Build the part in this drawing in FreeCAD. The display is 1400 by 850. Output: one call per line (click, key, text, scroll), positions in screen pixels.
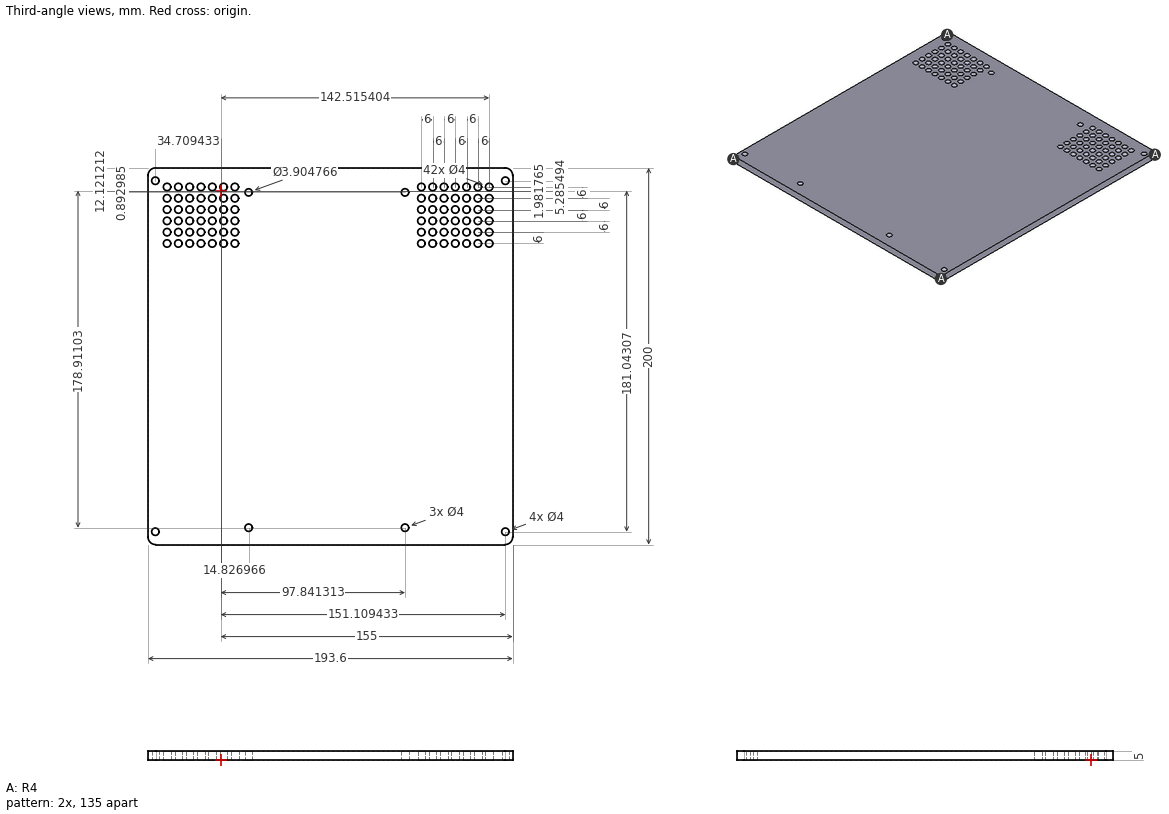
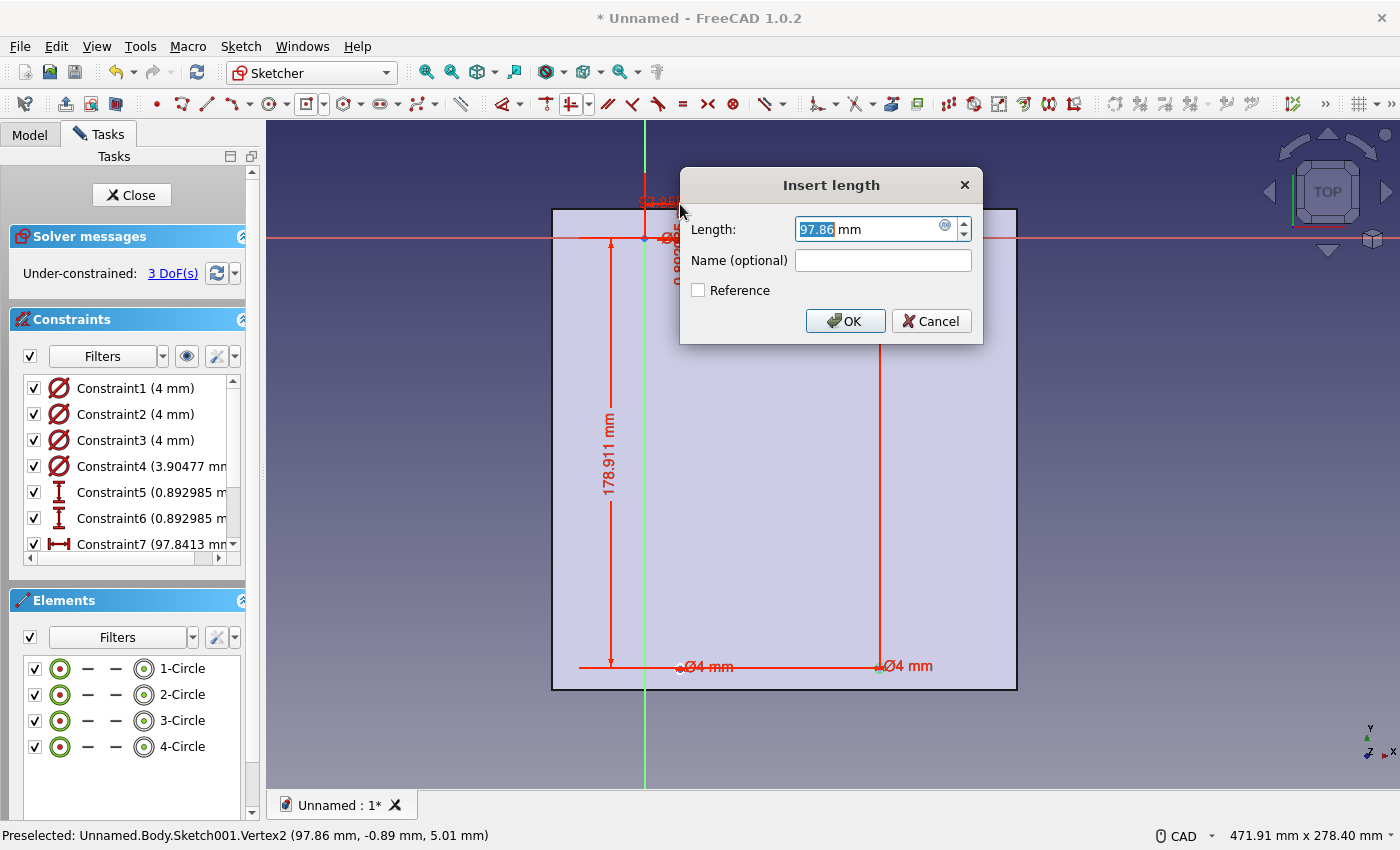
text(97.841313)
key(Return)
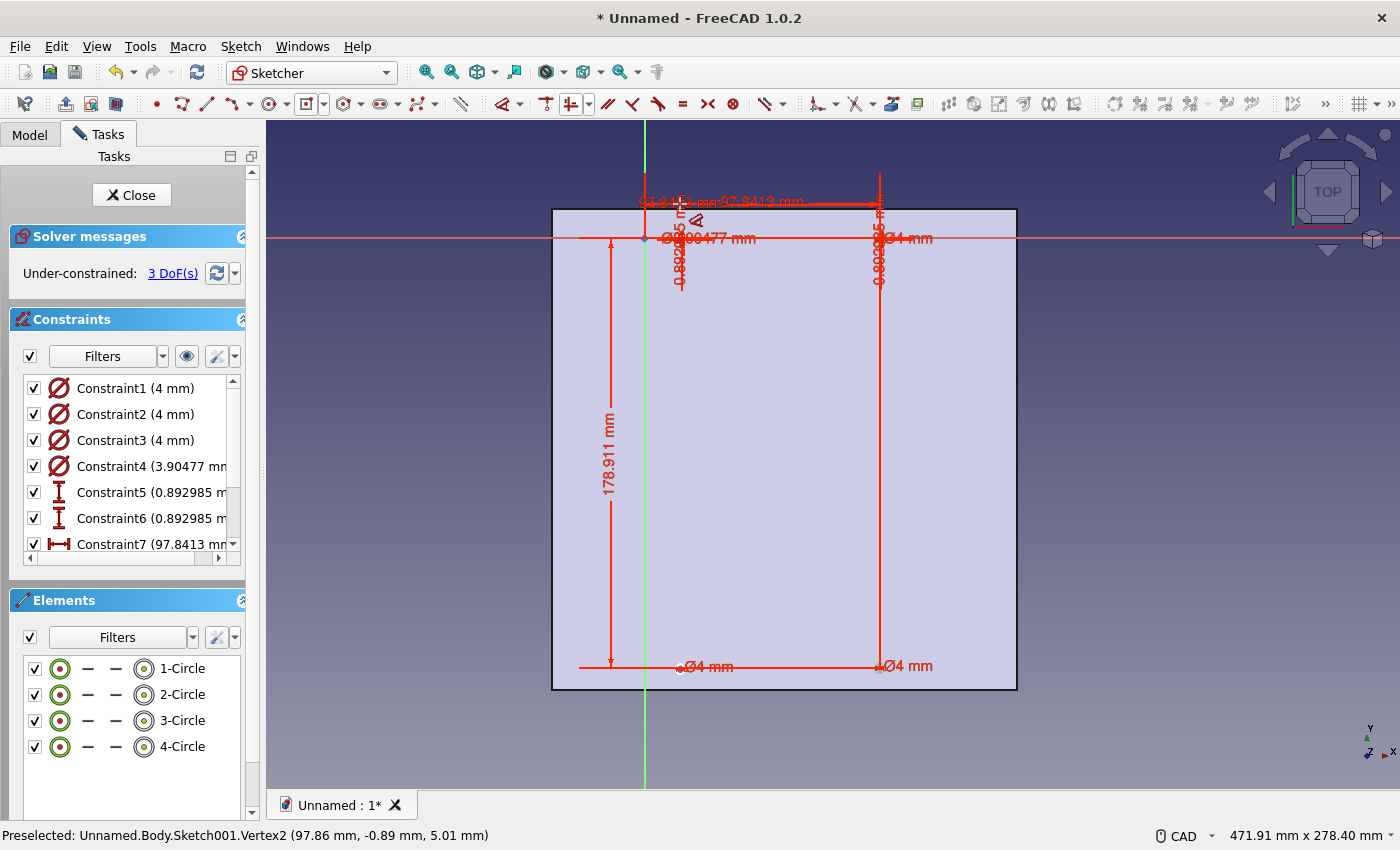
click(680, 669)
click(662, 703)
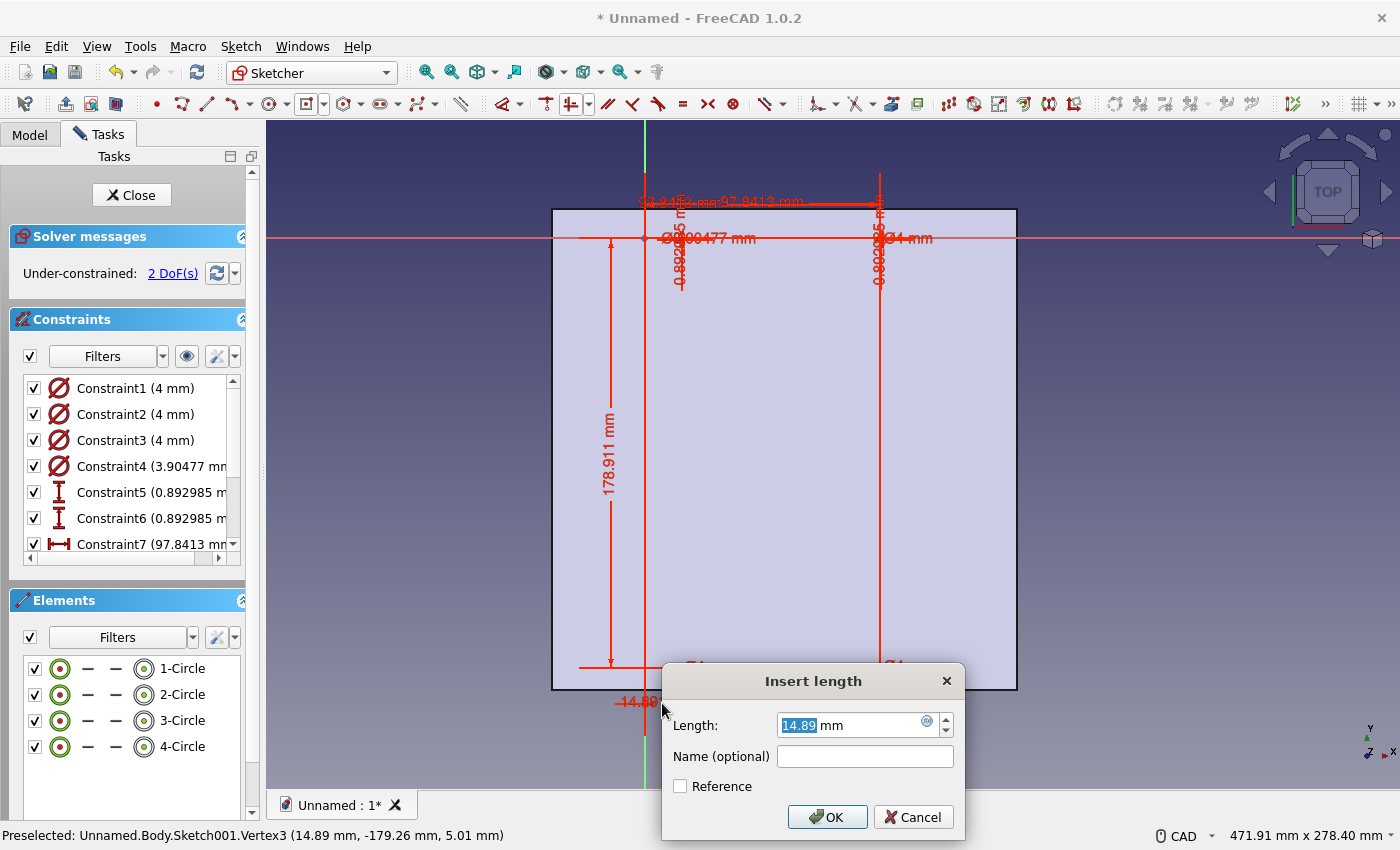
text(14.826966)
key(Return)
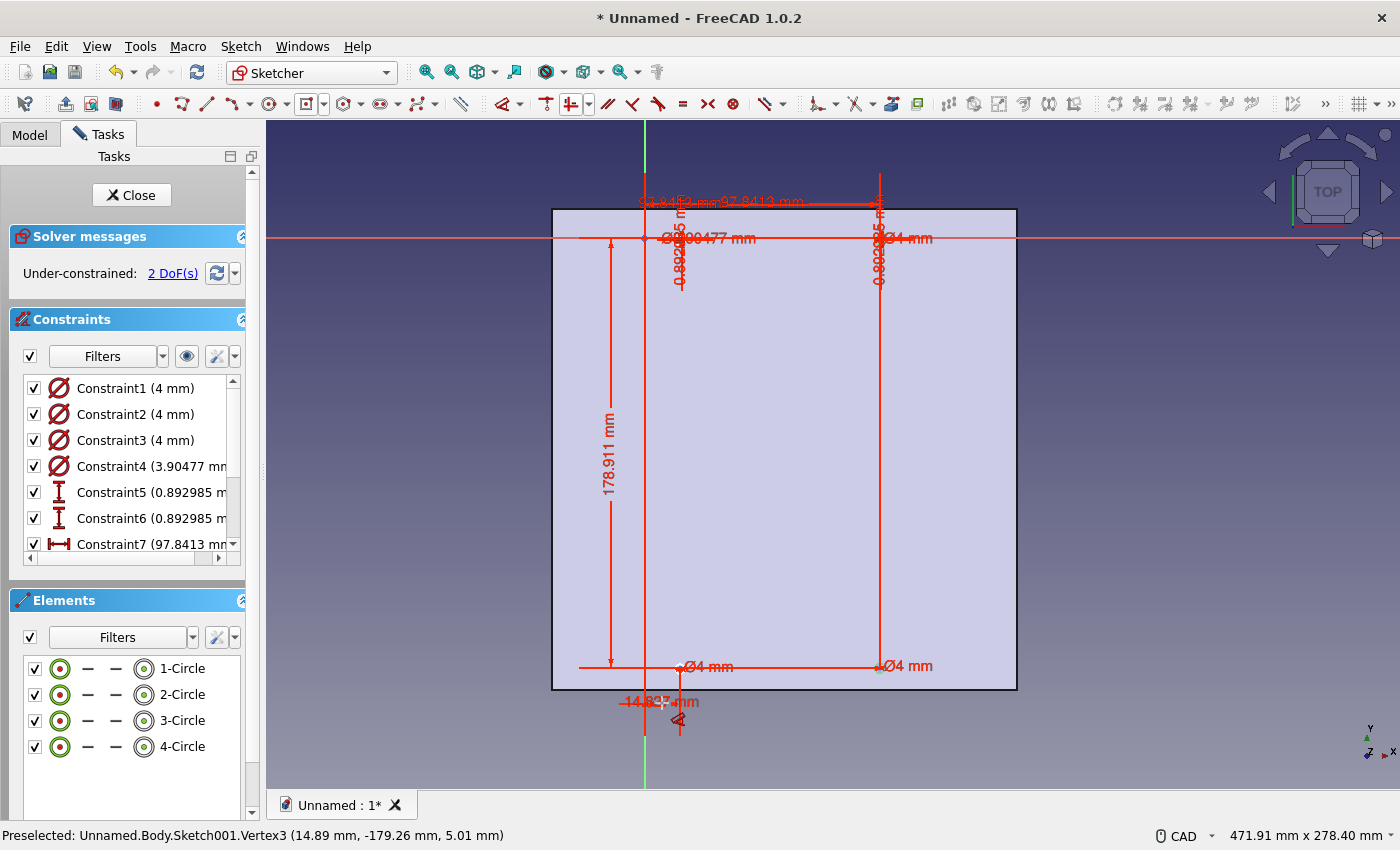
click(680, 669)
click(611, 355)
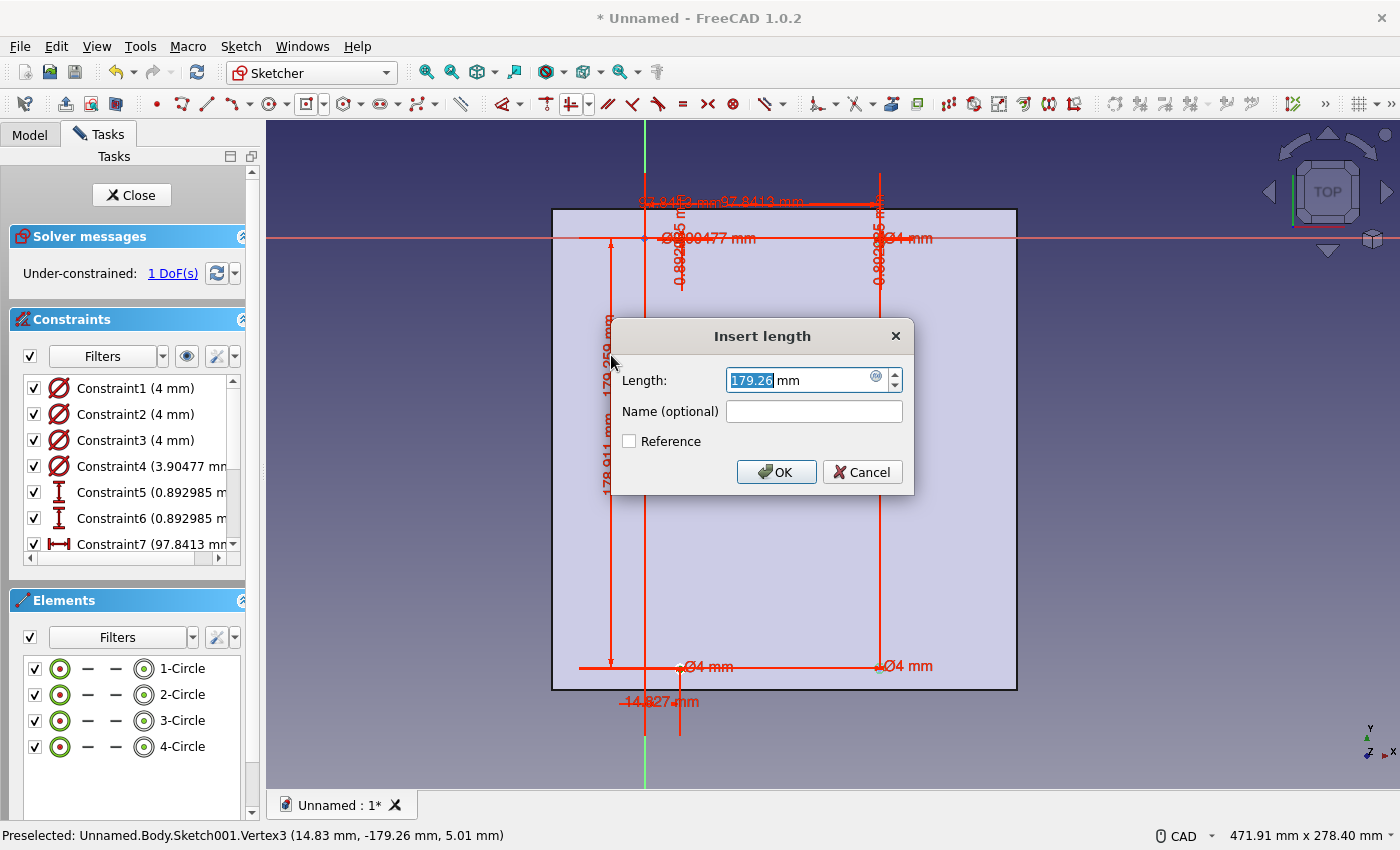
text(178.91103)
key(Return)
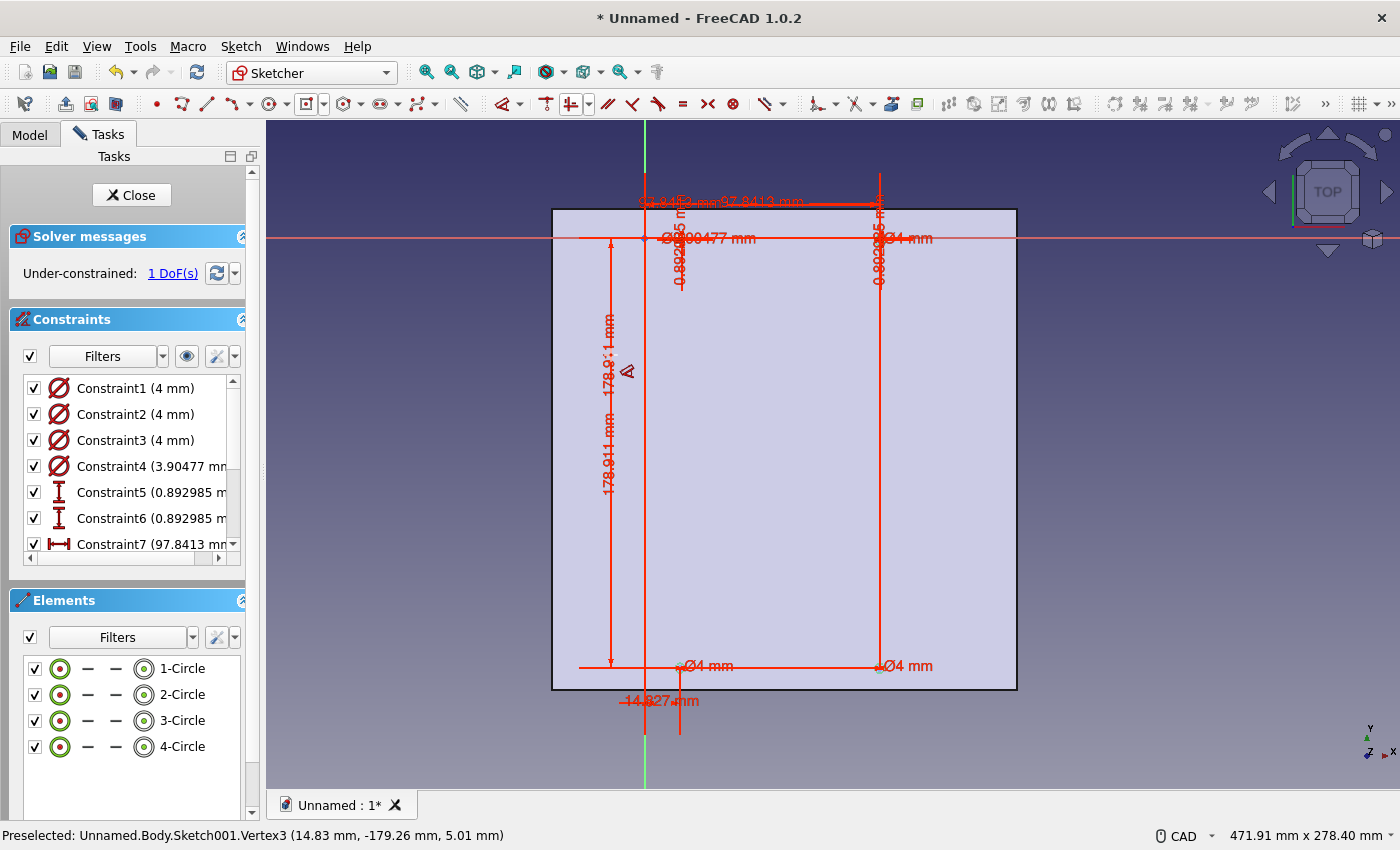
click(680, 240)
click(662, 274)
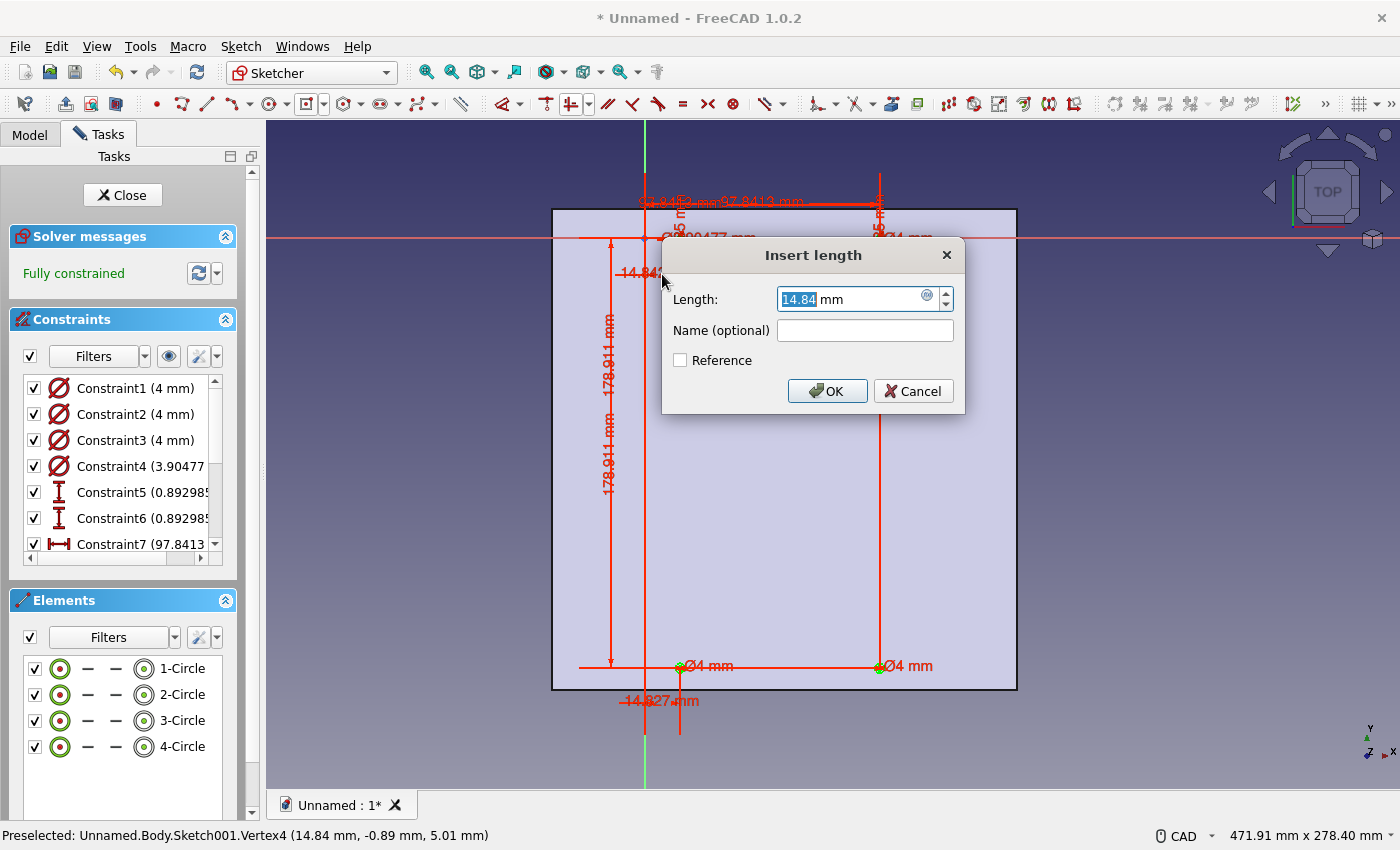
text(14.826966)
key(Return)
key(Escape)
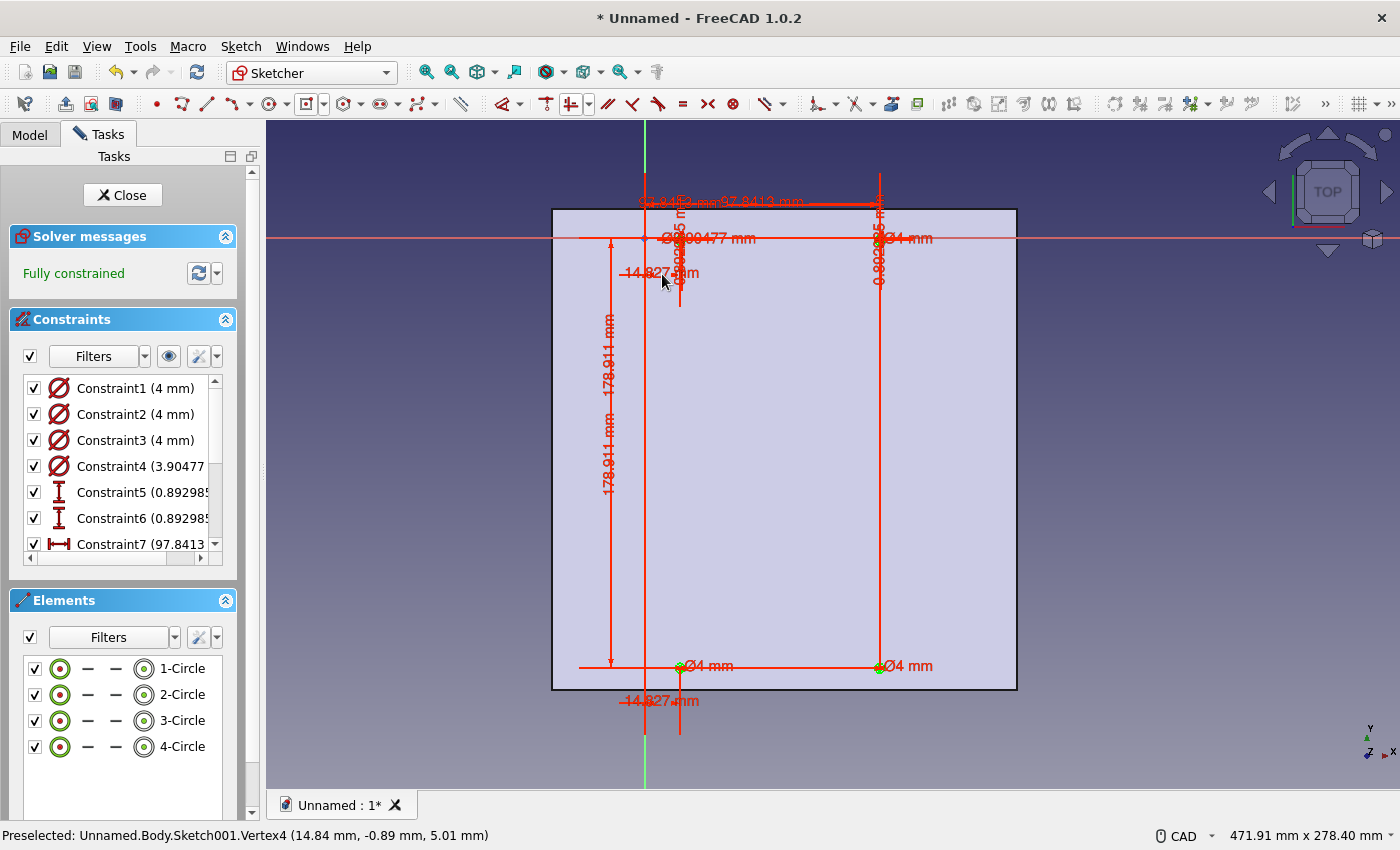
click(123, 195)